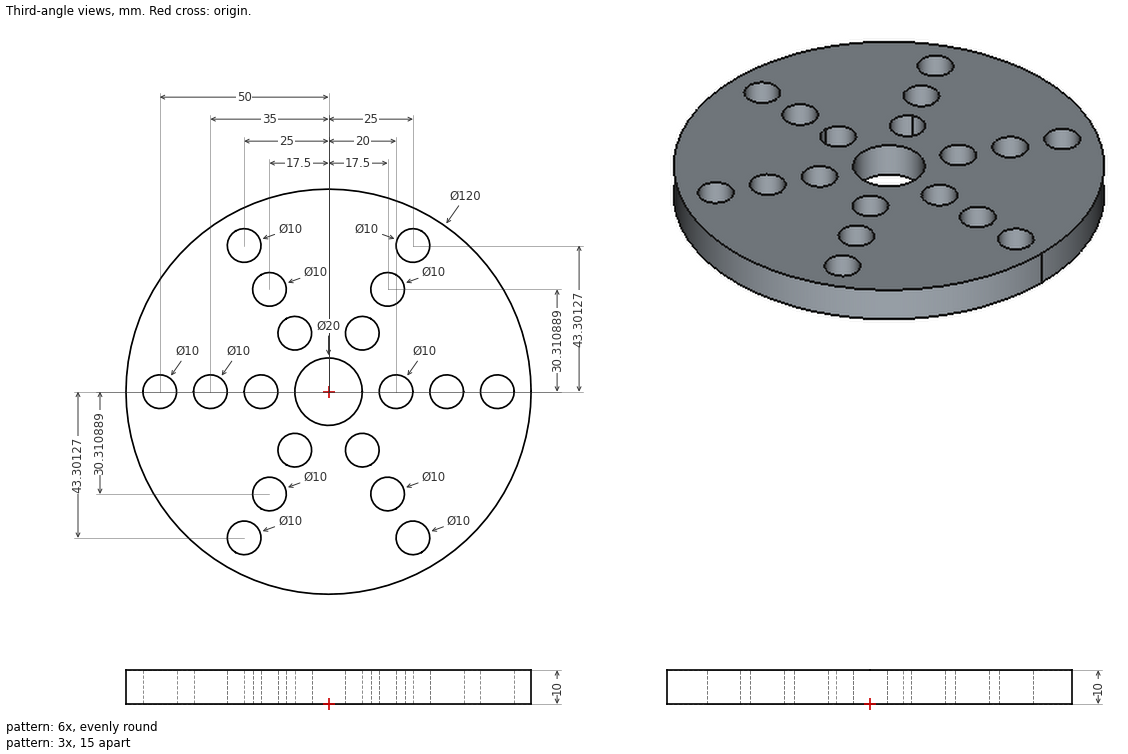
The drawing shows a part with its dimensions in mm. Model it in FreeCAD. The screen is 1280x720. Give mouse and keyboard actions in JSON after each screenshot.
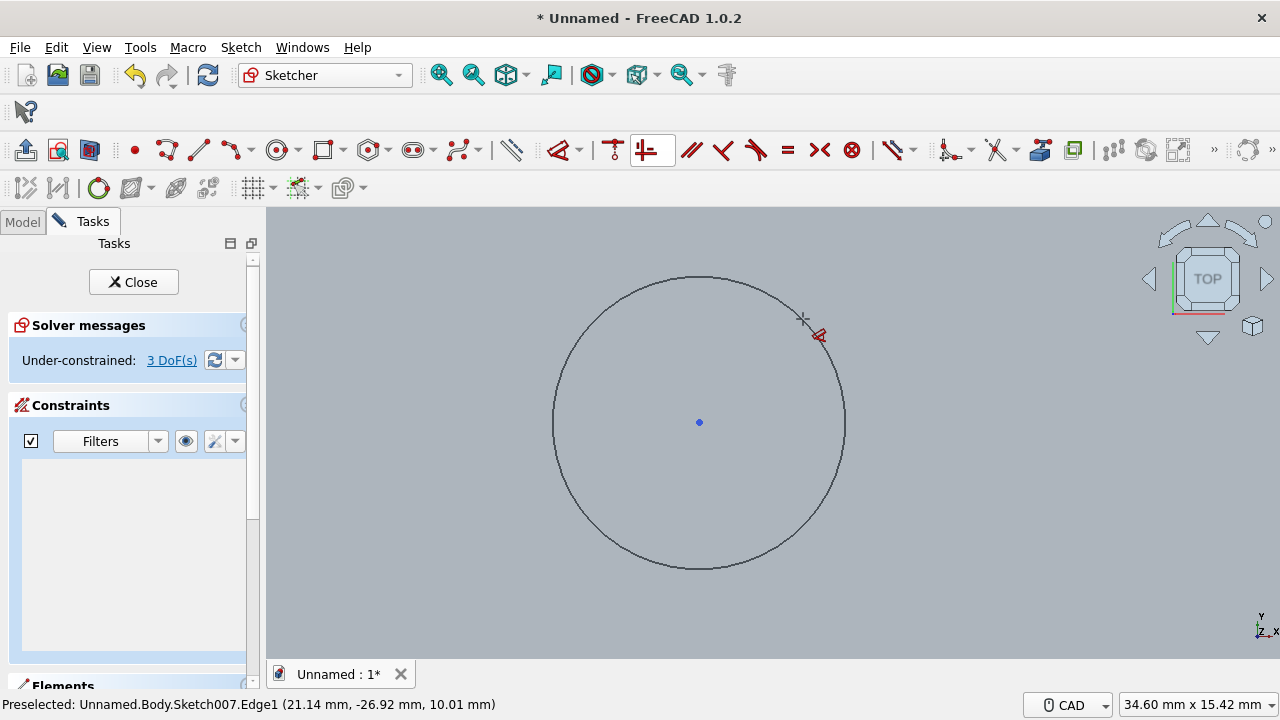
{"action": "left_click", "coordinate": [802, 319]}
{"action": "left_click", "coordinate": [825, 296]}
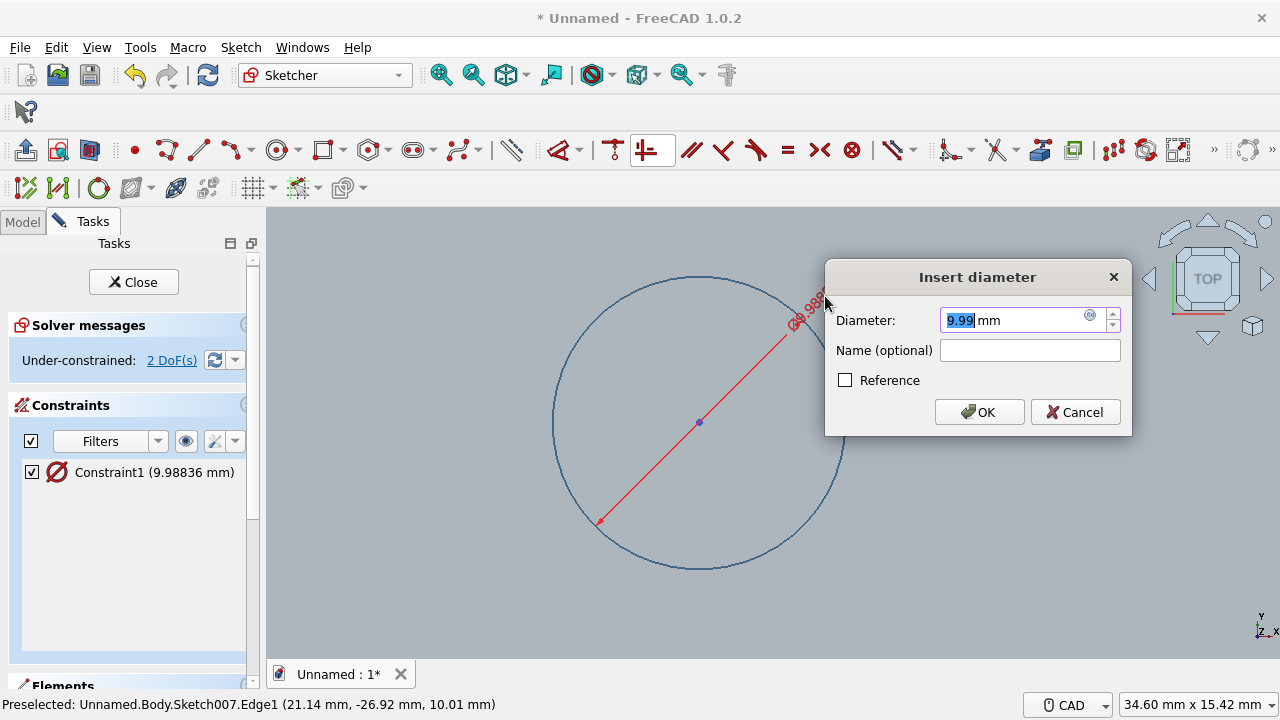
{"action": "type", "text": "10"}
{"action": "key", "text": "Return"}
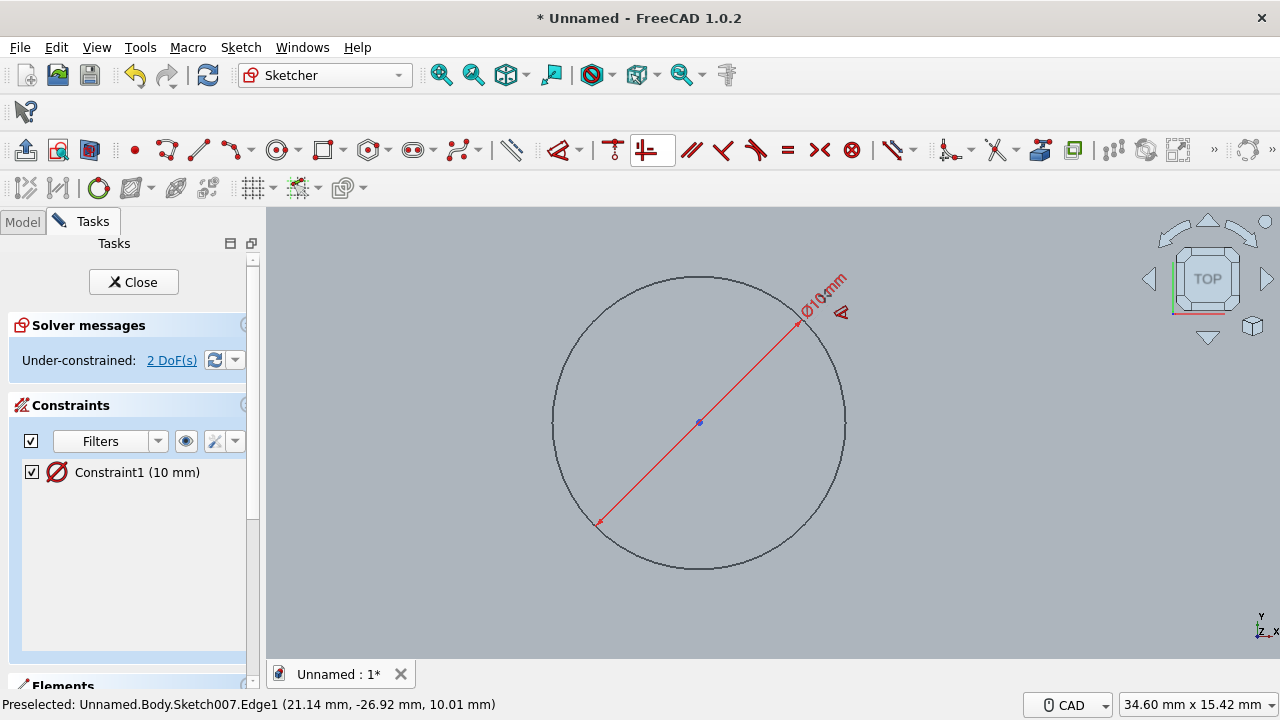
{"action": "left_click", "coordinate": [699, 423]}
{"action": "left_click", "coordinate": [496, 457]}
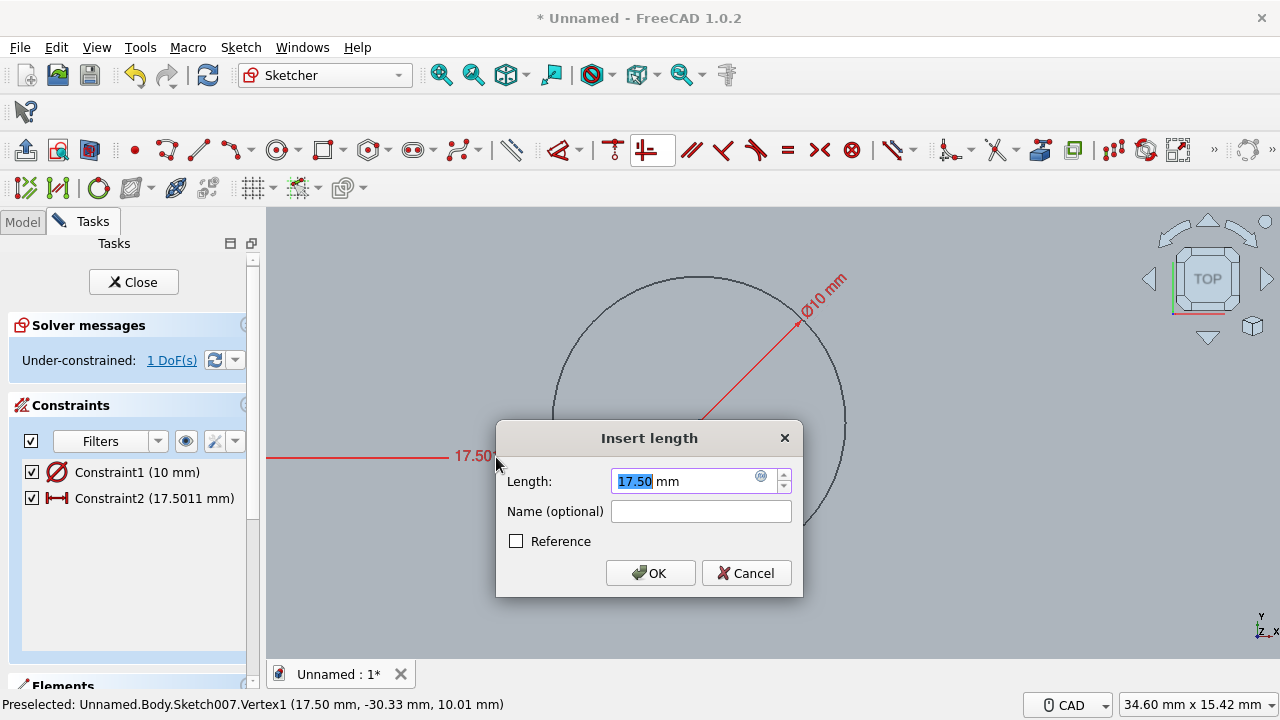
{"action": "type", "text": "17.5"}
{"action": "key", "text": "Return"}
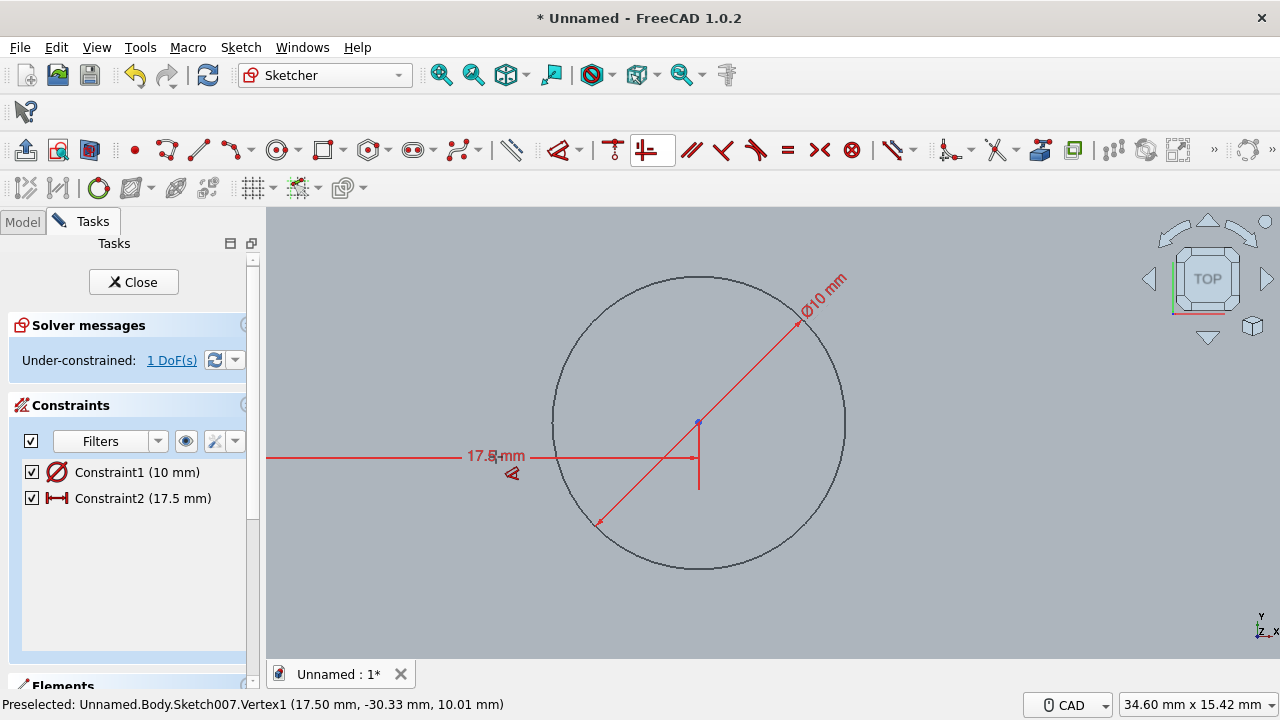
{"action": "left_click", "coordinate": [699, 423]}
{"action": "left_click", "coordinate": [733, 329]}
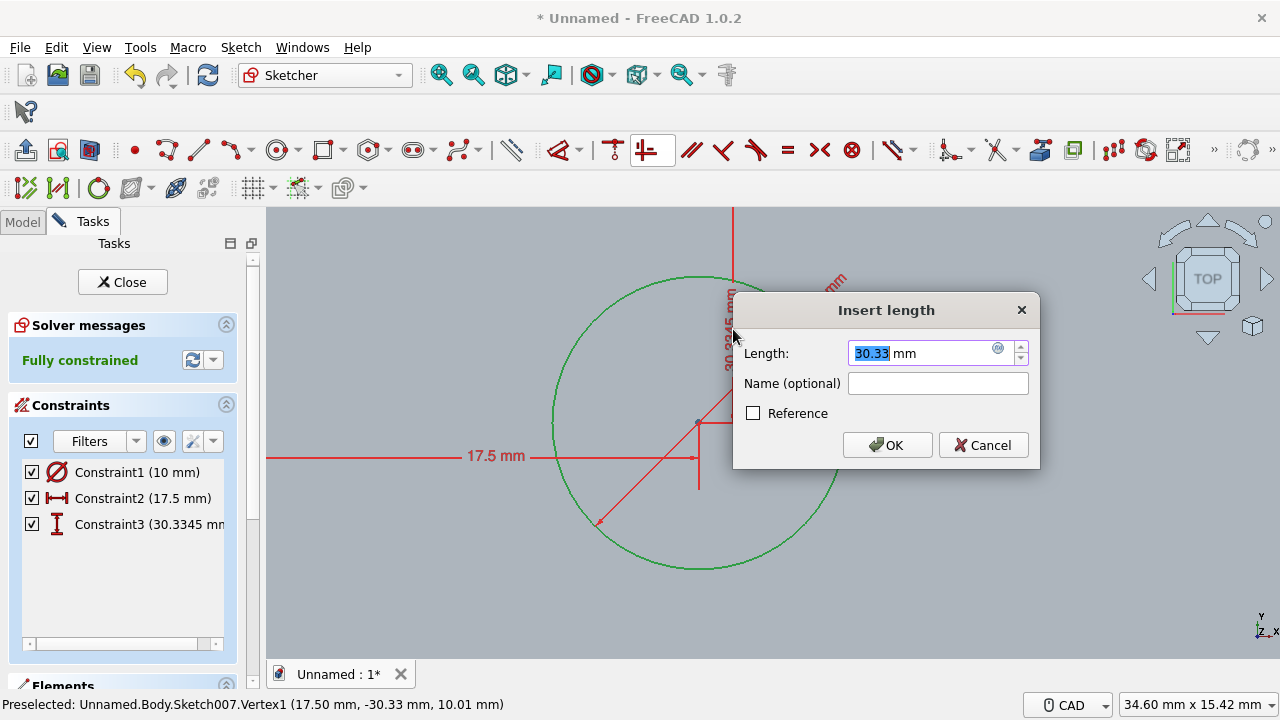
{"action": "type", "text": "30.310889"}
{"action": "key", "text": "Return"}
{"action": "key", "text": "Escape"}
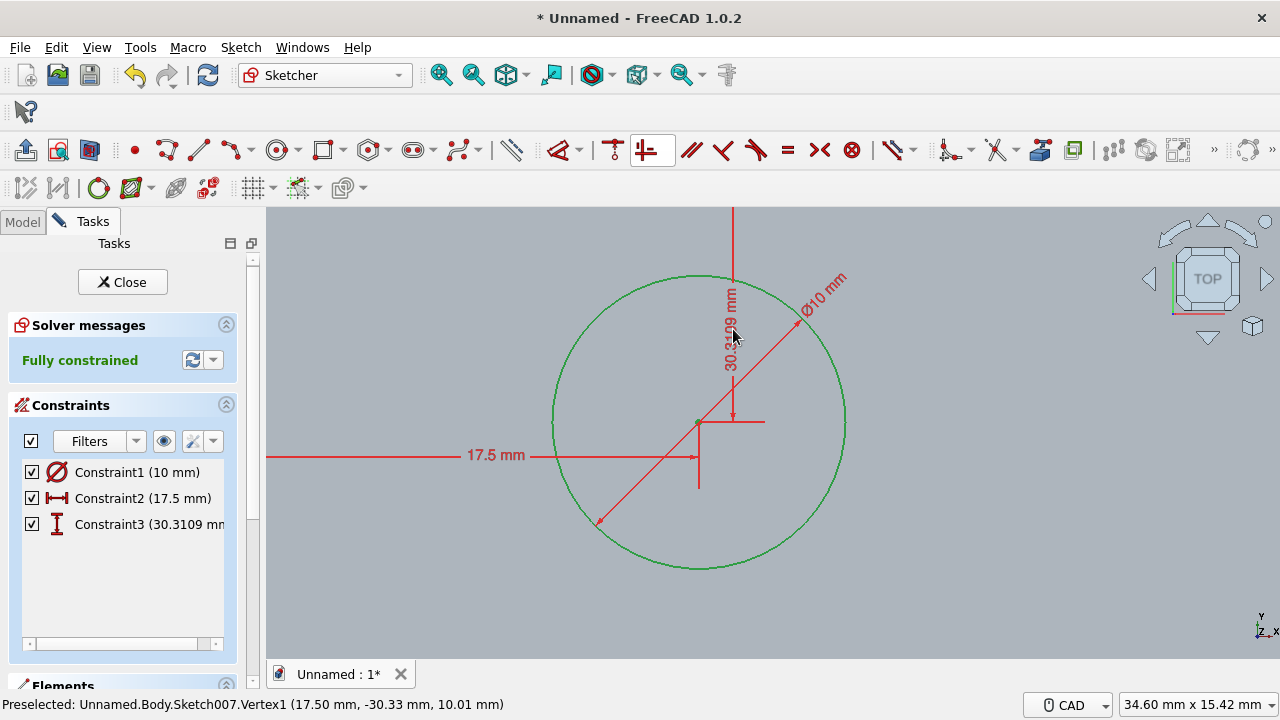
{"action": "left_click", "coordinate": [123, 282]}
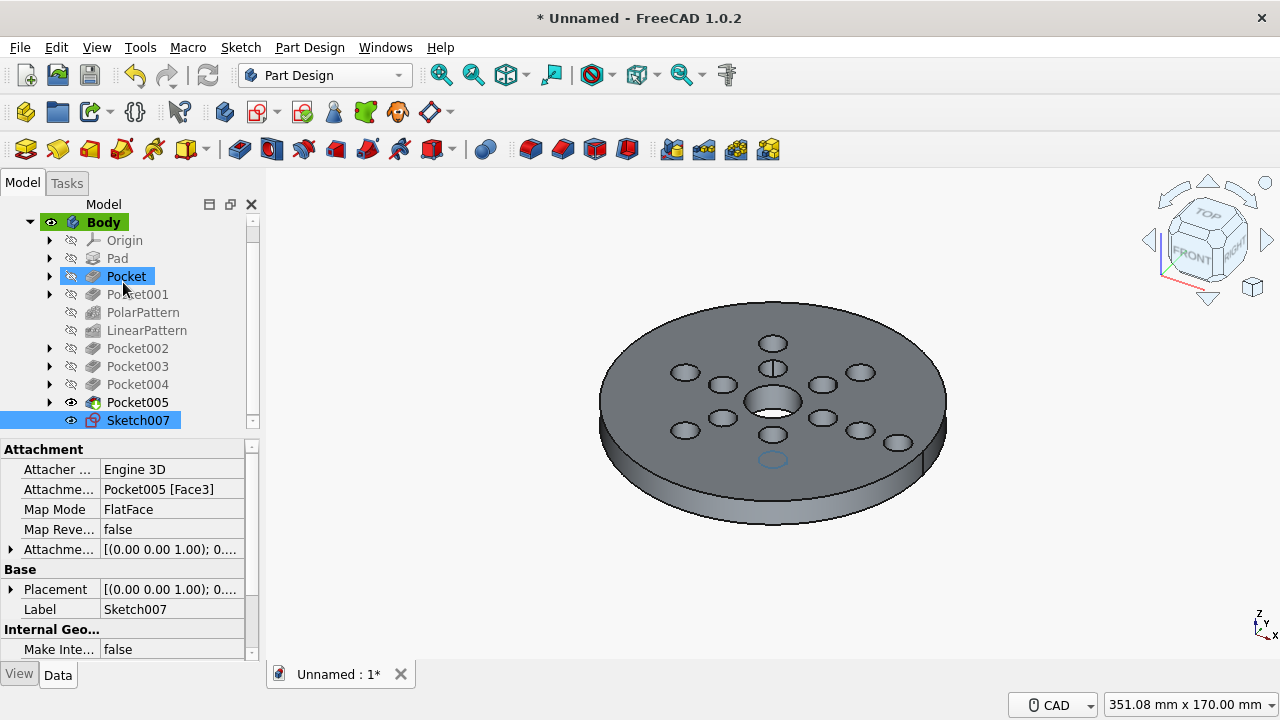
{"action": "left_click", "coordinate": [240, 150]}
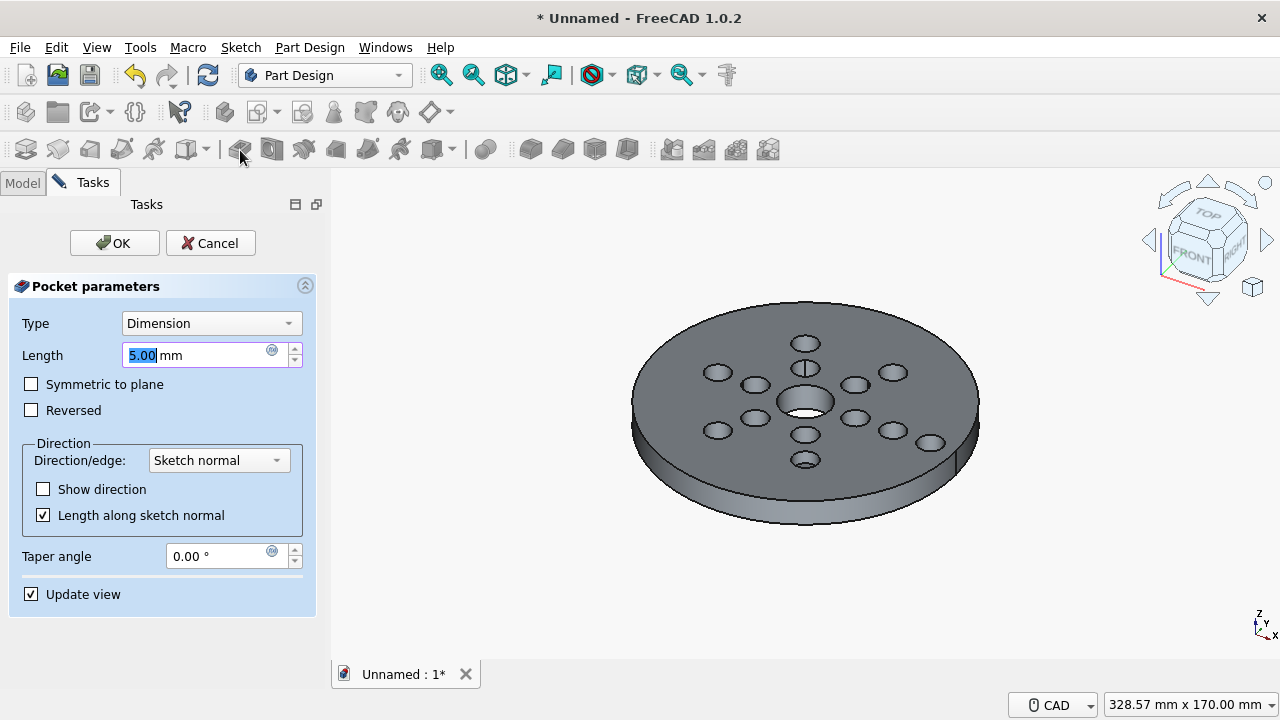
{"action": "type", "text": "10"}
{"action": "key", "text": "Tab"}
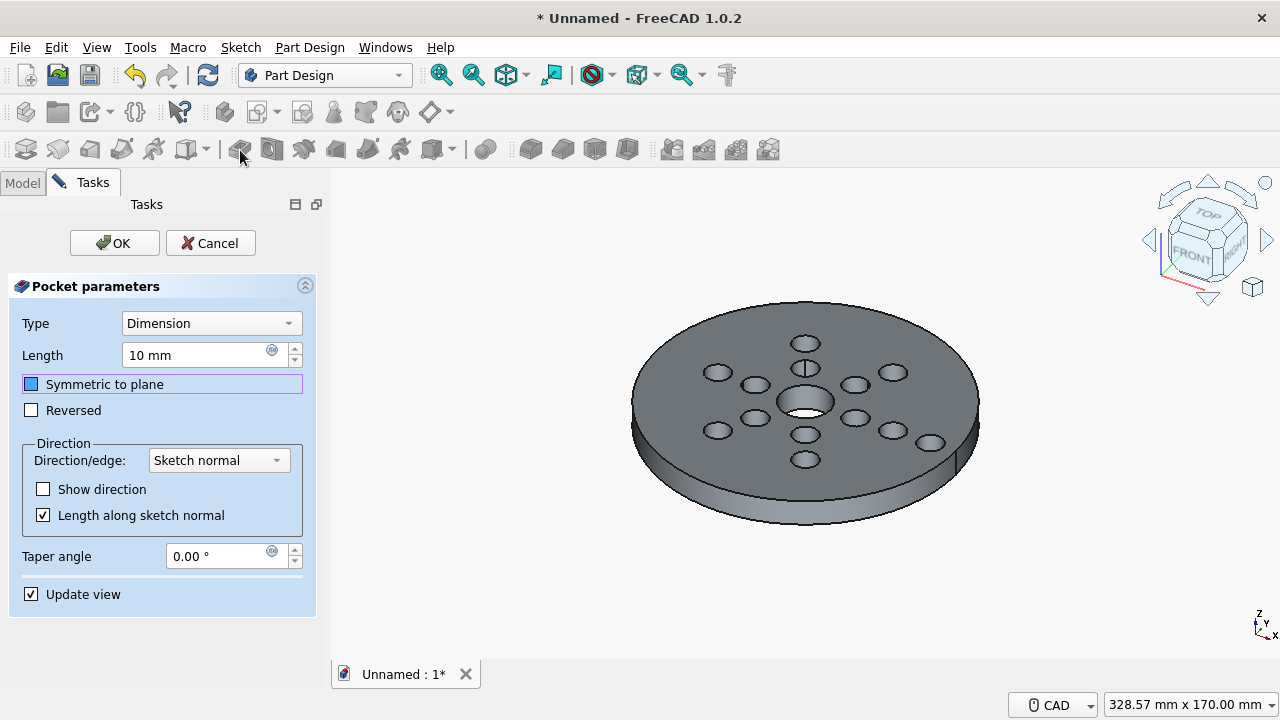
{"action": "left_click", "coordinate": [115, 243]}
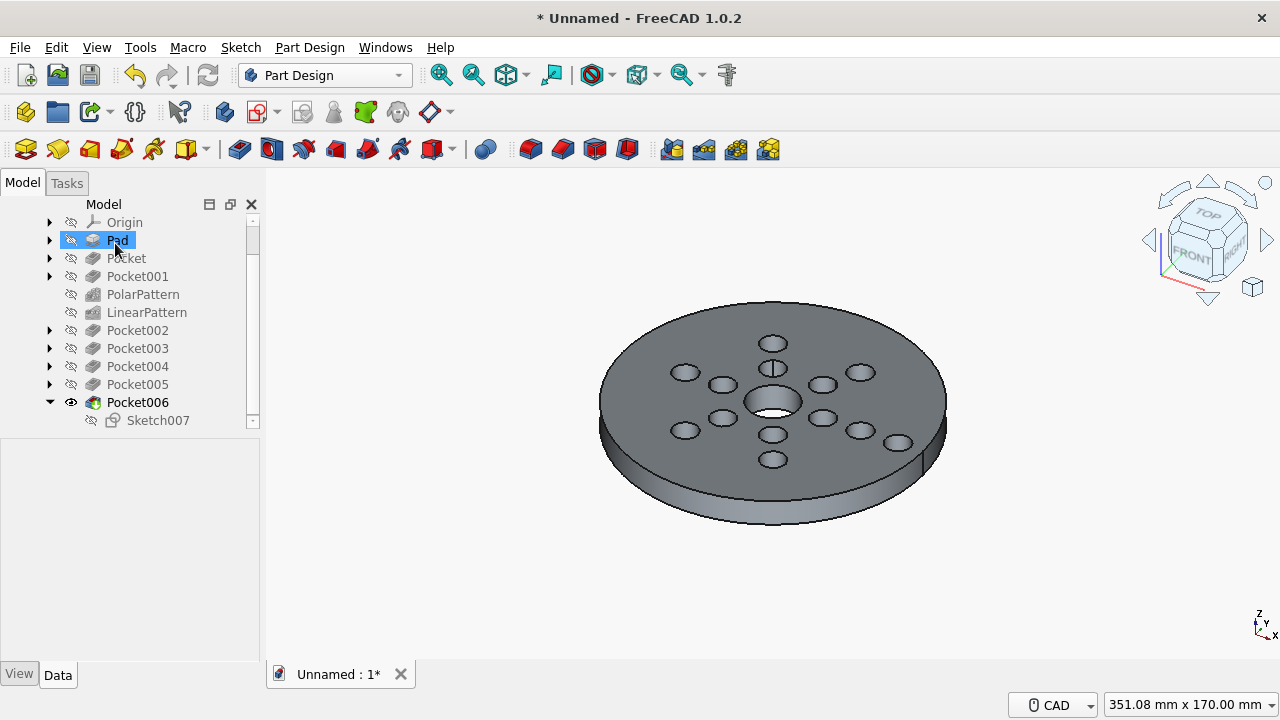
{"action": "left_click", "coordinate": [823, 351]}